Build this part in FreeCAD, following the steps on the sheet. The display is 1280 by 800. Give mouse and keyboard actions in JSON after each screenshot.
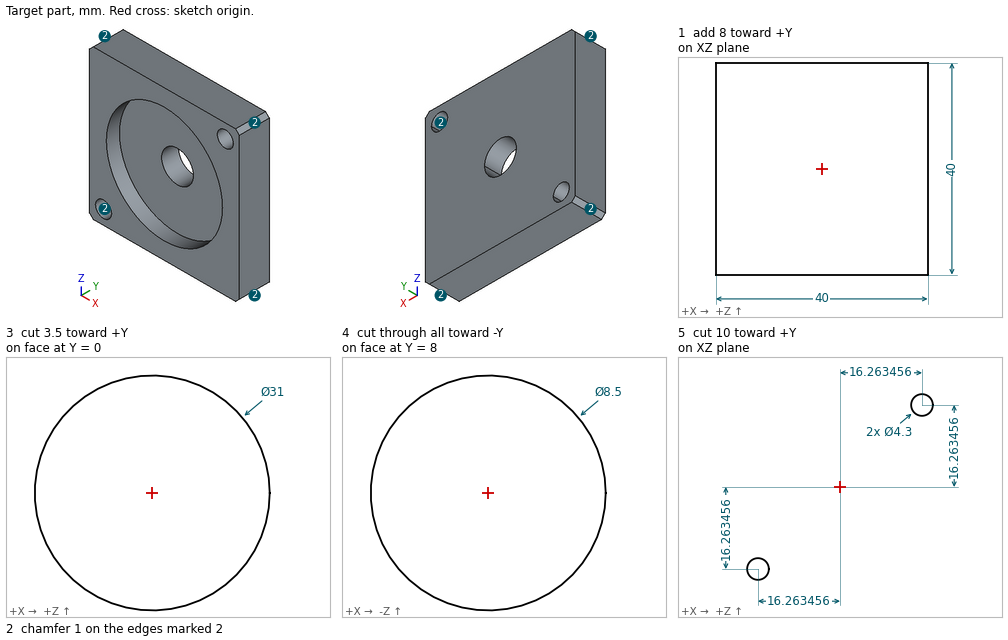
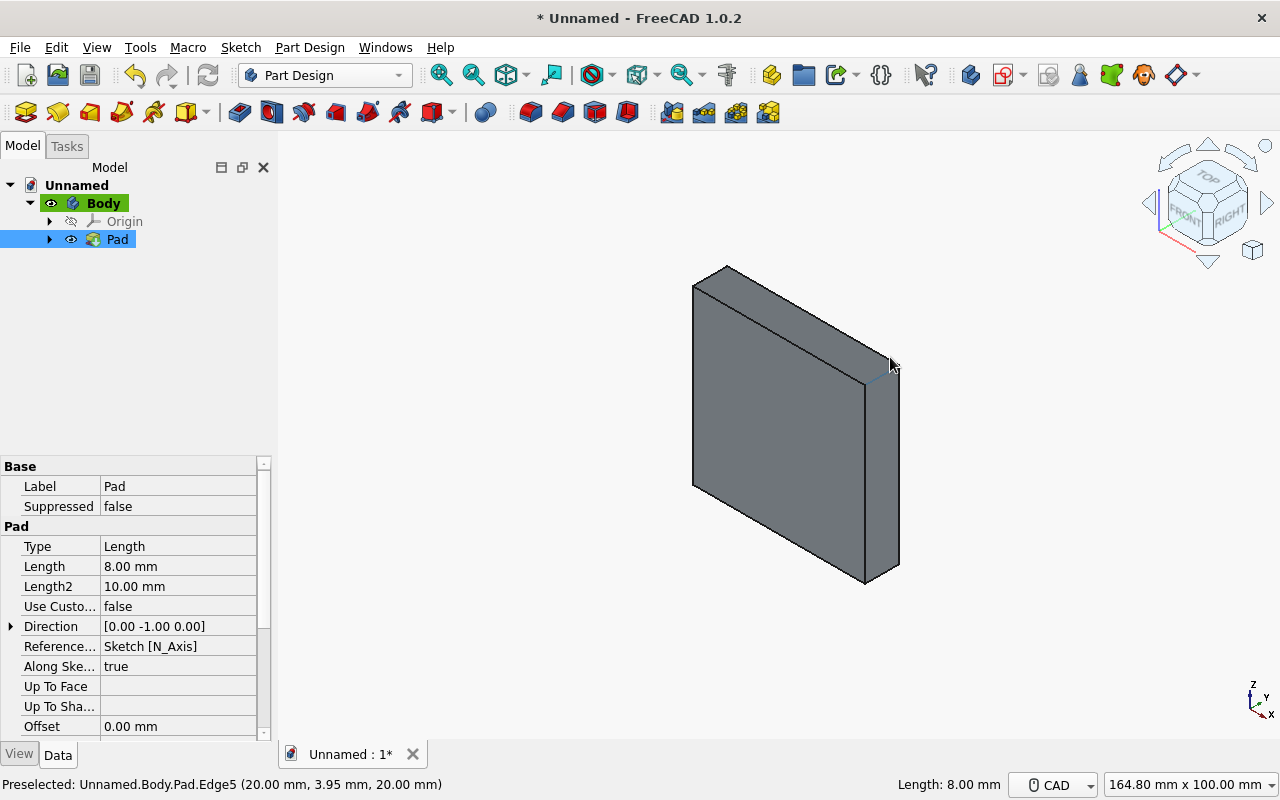
{"action": "key", "text": "2"}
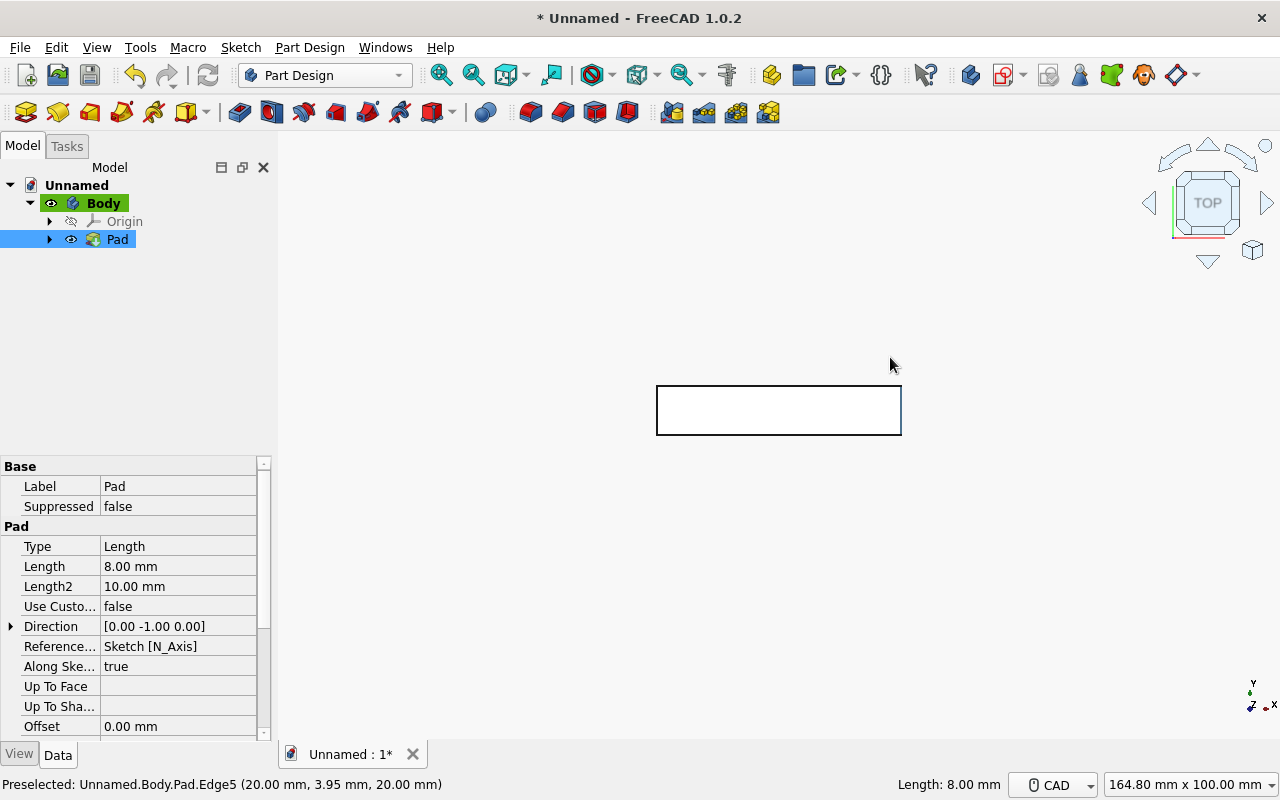
{"action": "left_click", "coordinate": [442, 76]}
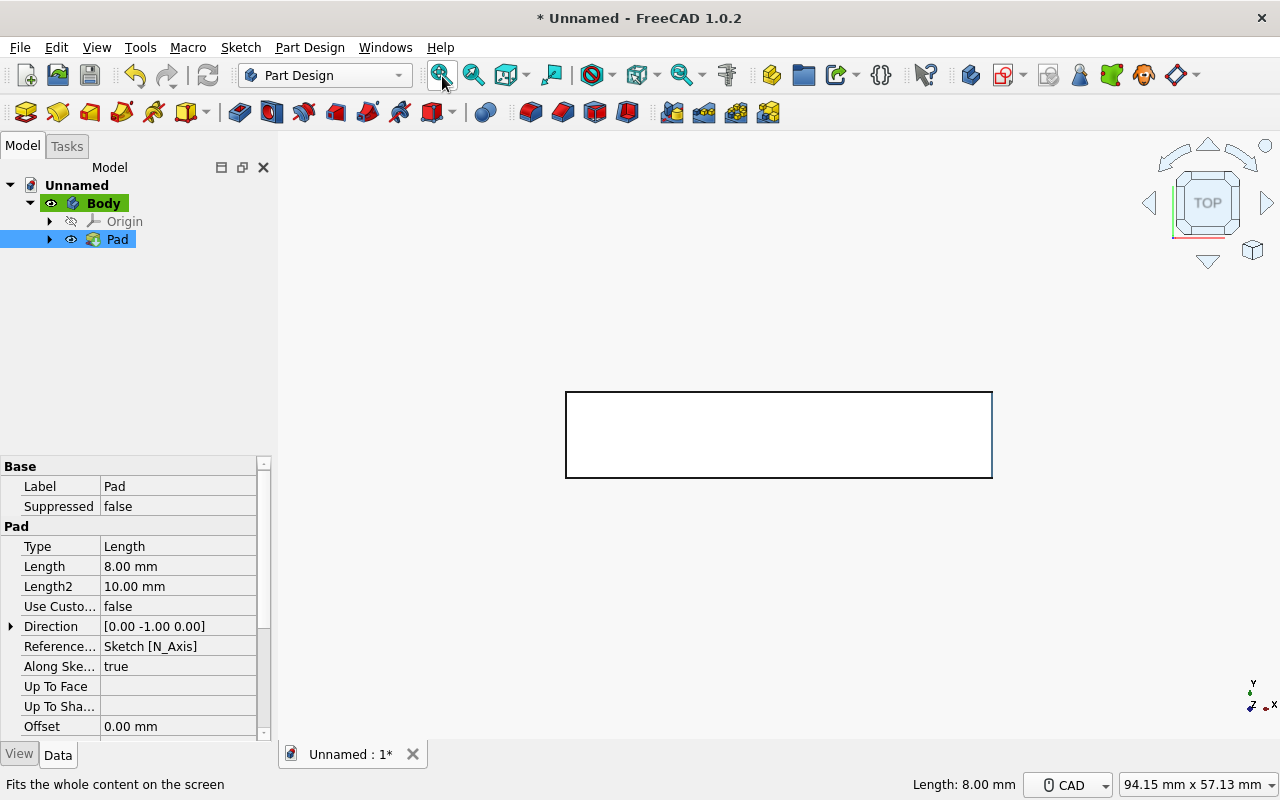
{"action": "left_click", "coordinate": [566, 434], "text": "ctrl"}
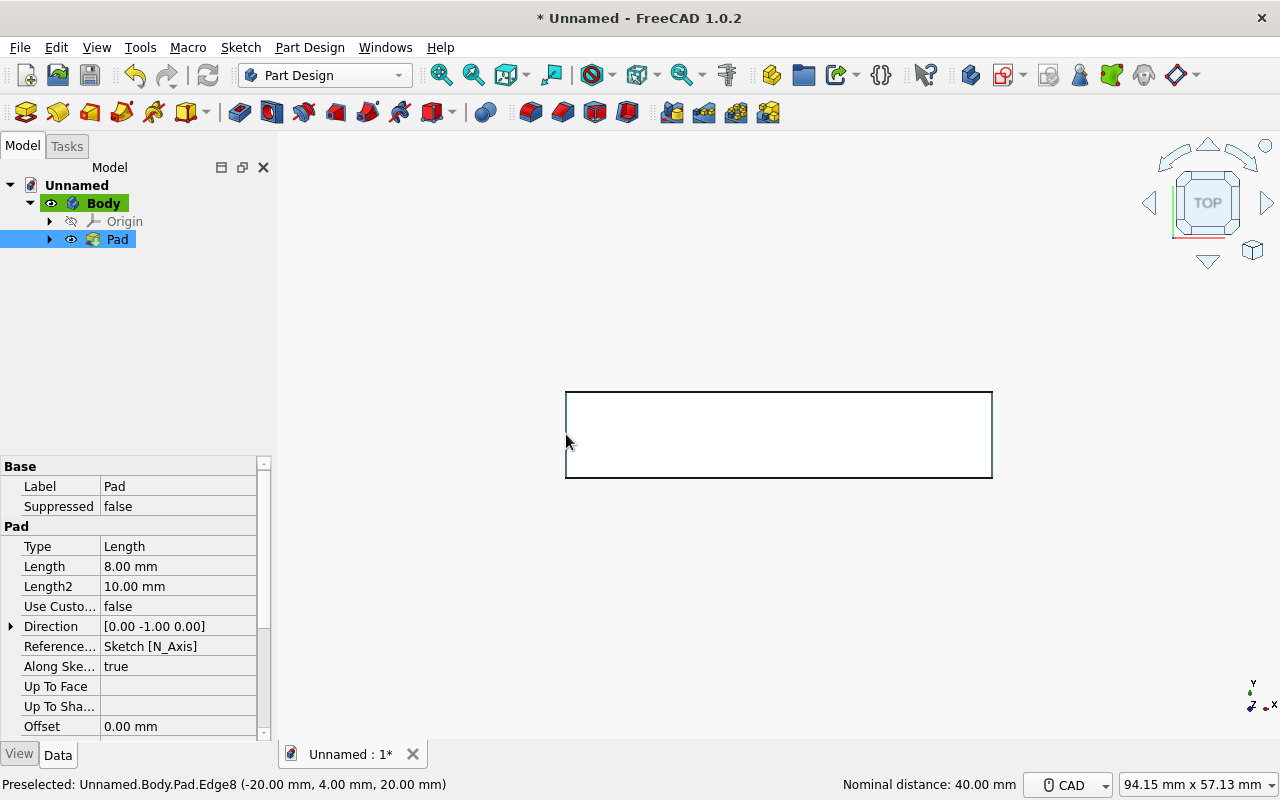
{"action": "key", "text": "1"}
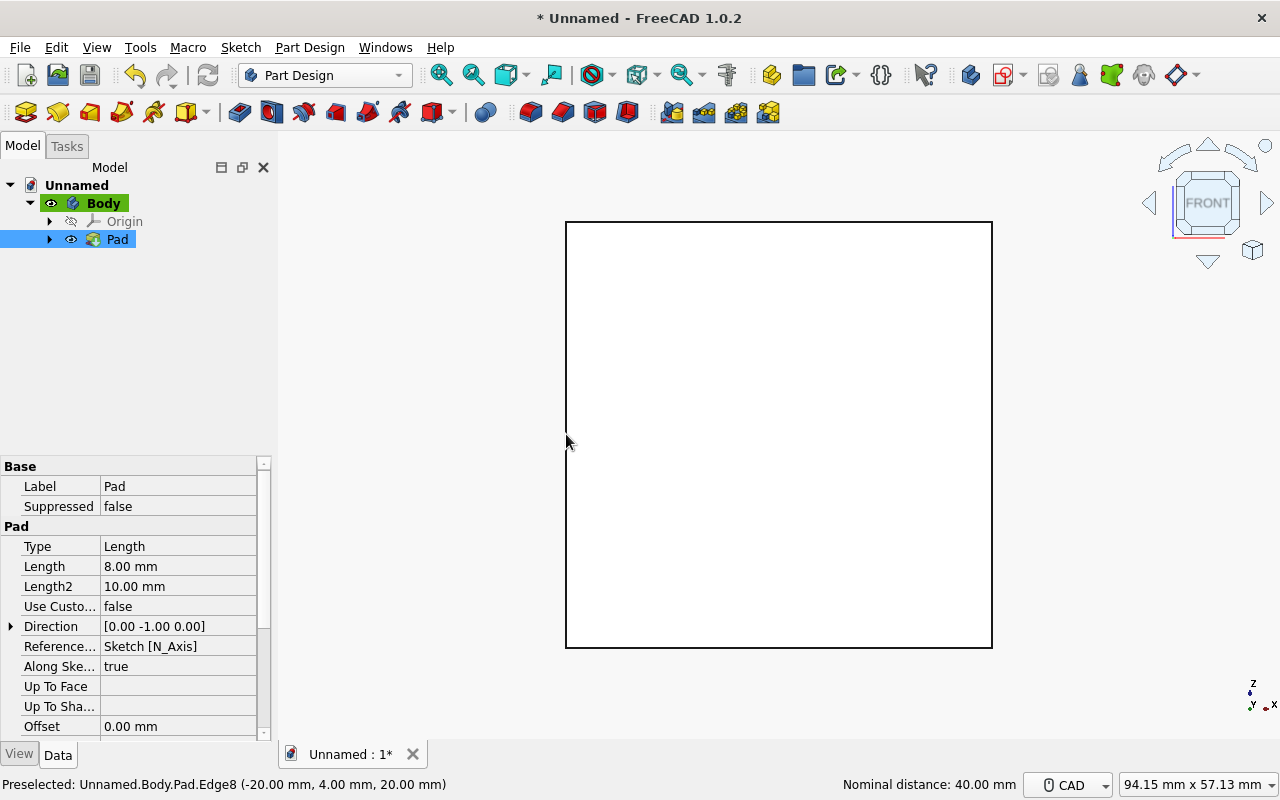
{"action": "key", "text": "3"}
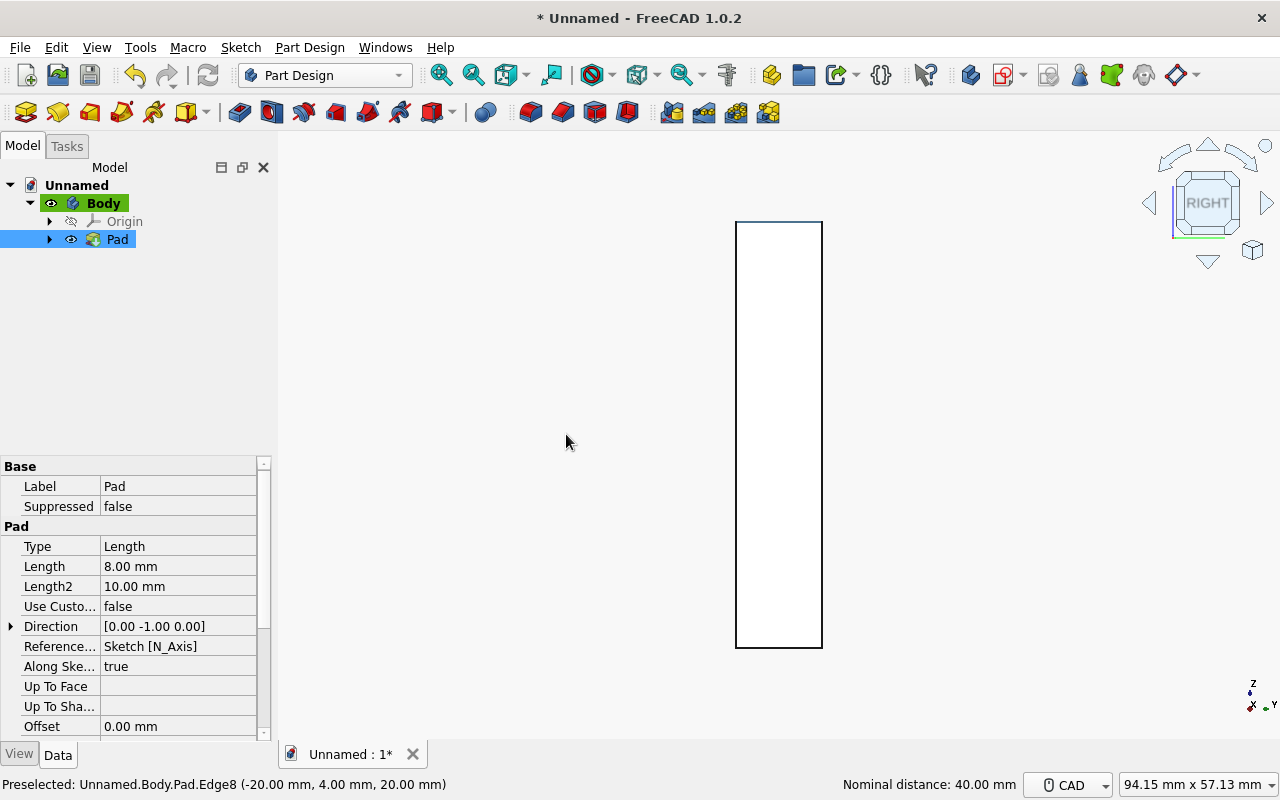
{"action": "left_click", "coordinate": [779, 647], "text": "ctrl"}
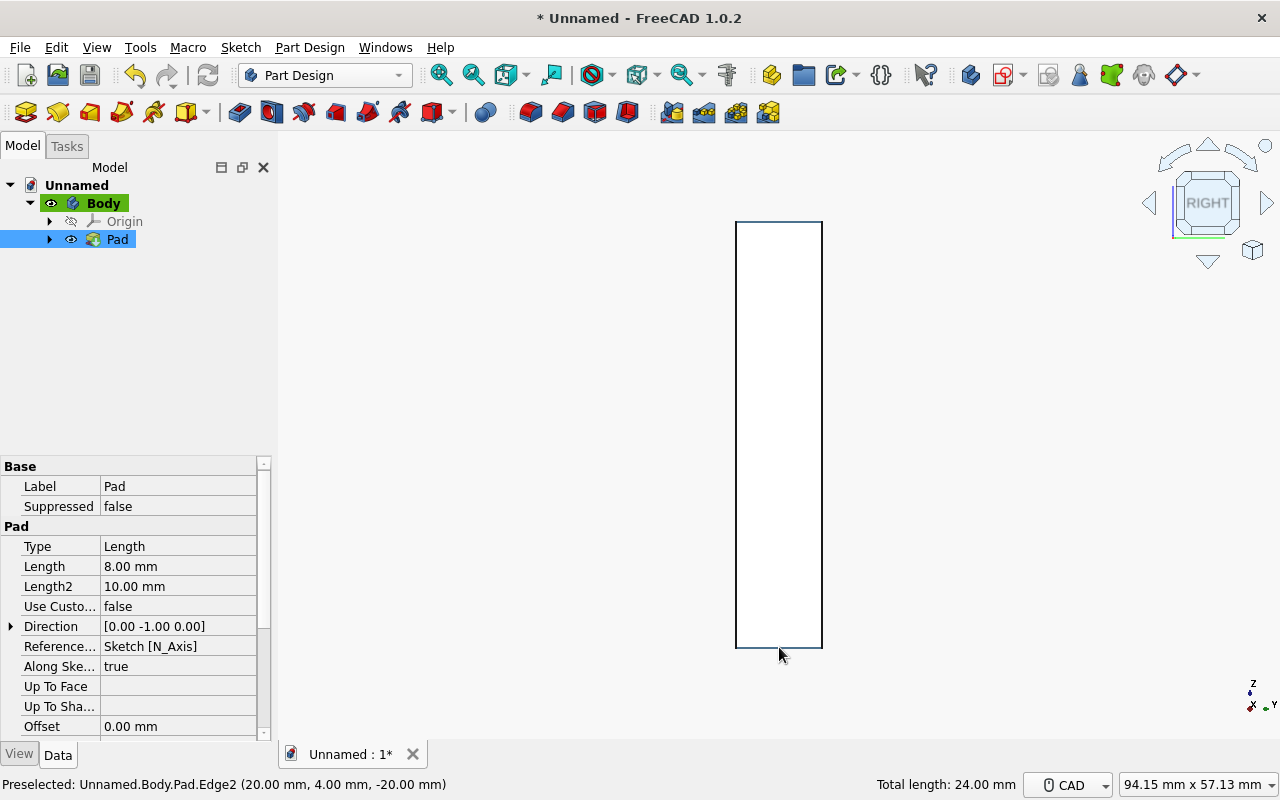
{"action": "key", "text": "5"}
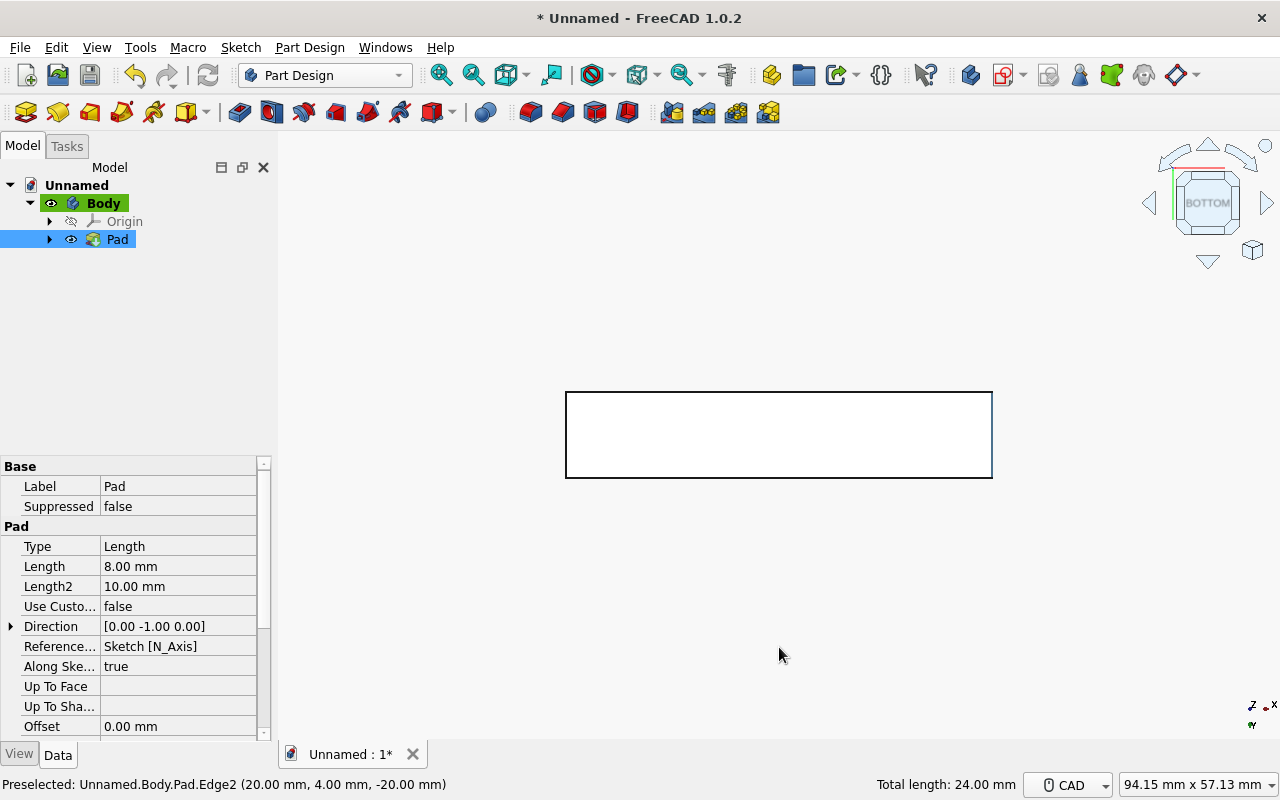
{"action": "left_click", "coordinate": [442, 76]}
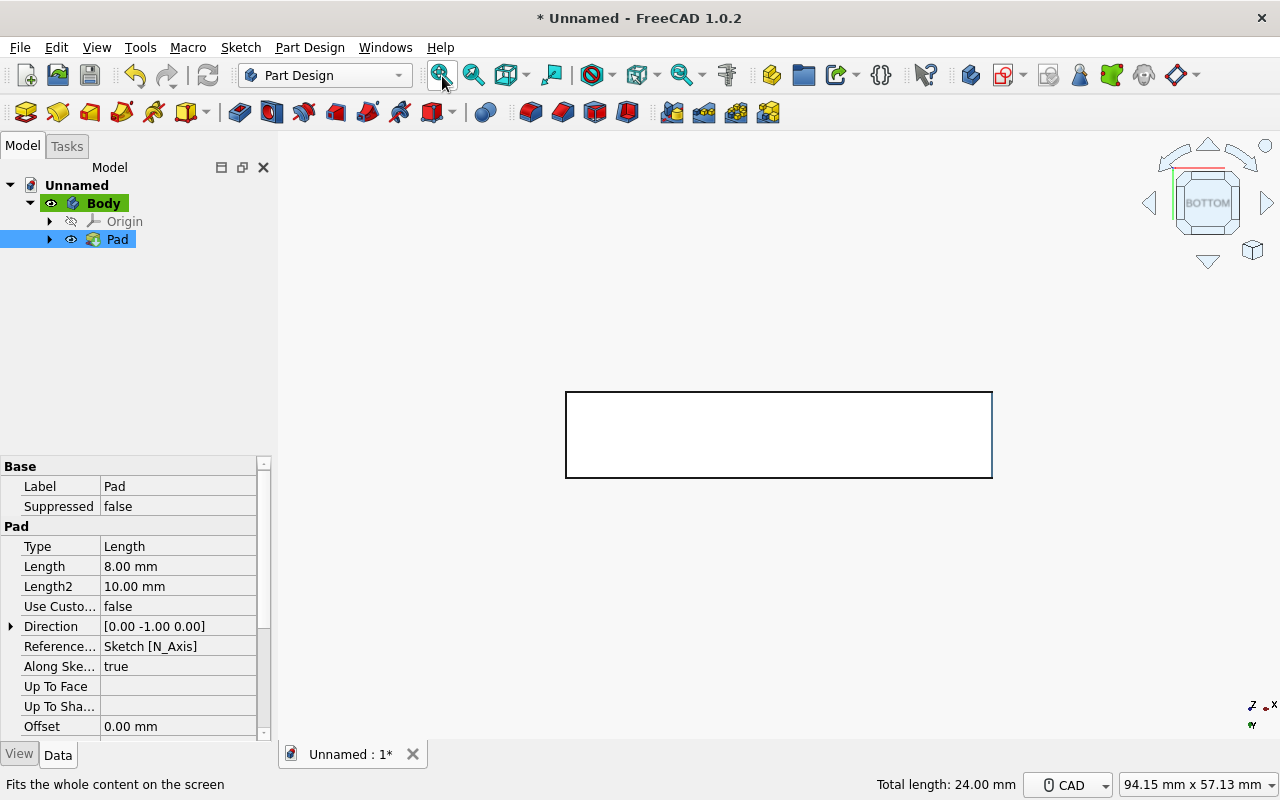
{"action": "left_click", "coordinate": [566, 434], "text": "ctrl"}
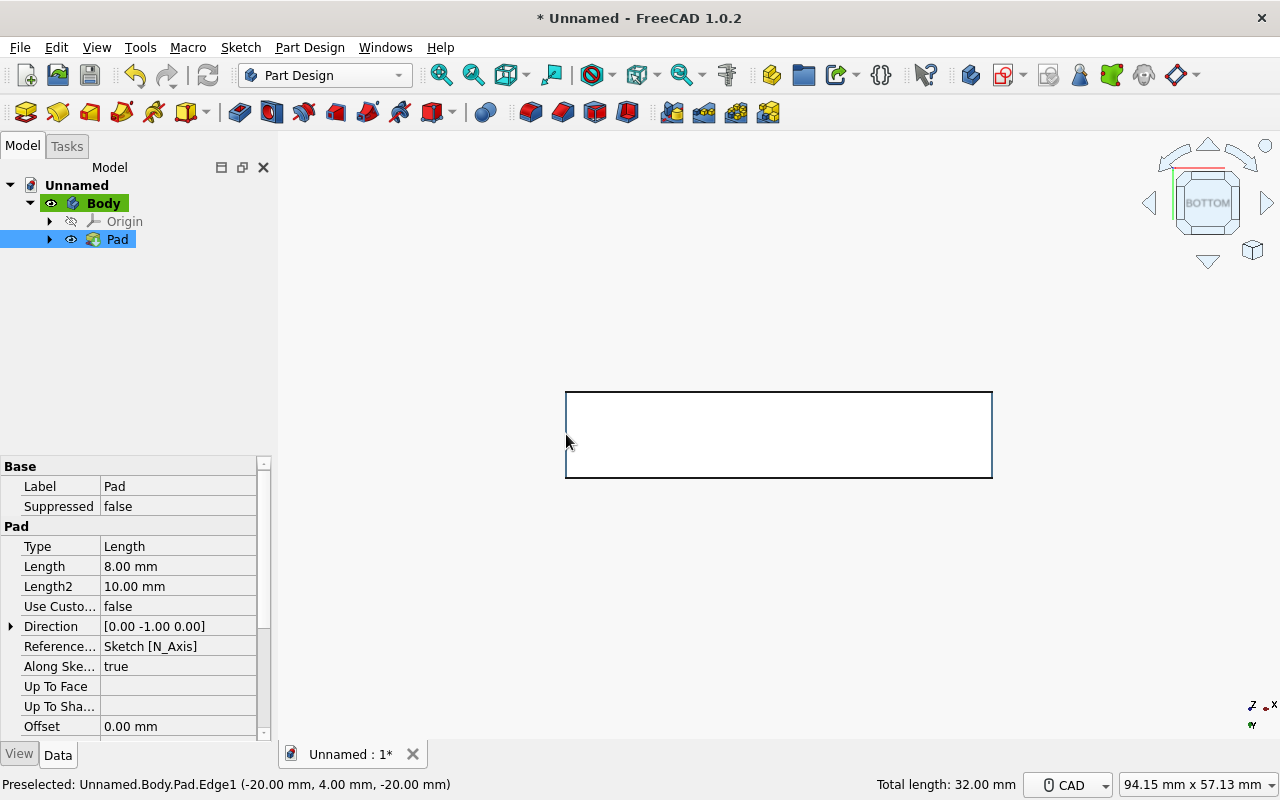
{"action": "left_click", "coordinate": [564, 112]}